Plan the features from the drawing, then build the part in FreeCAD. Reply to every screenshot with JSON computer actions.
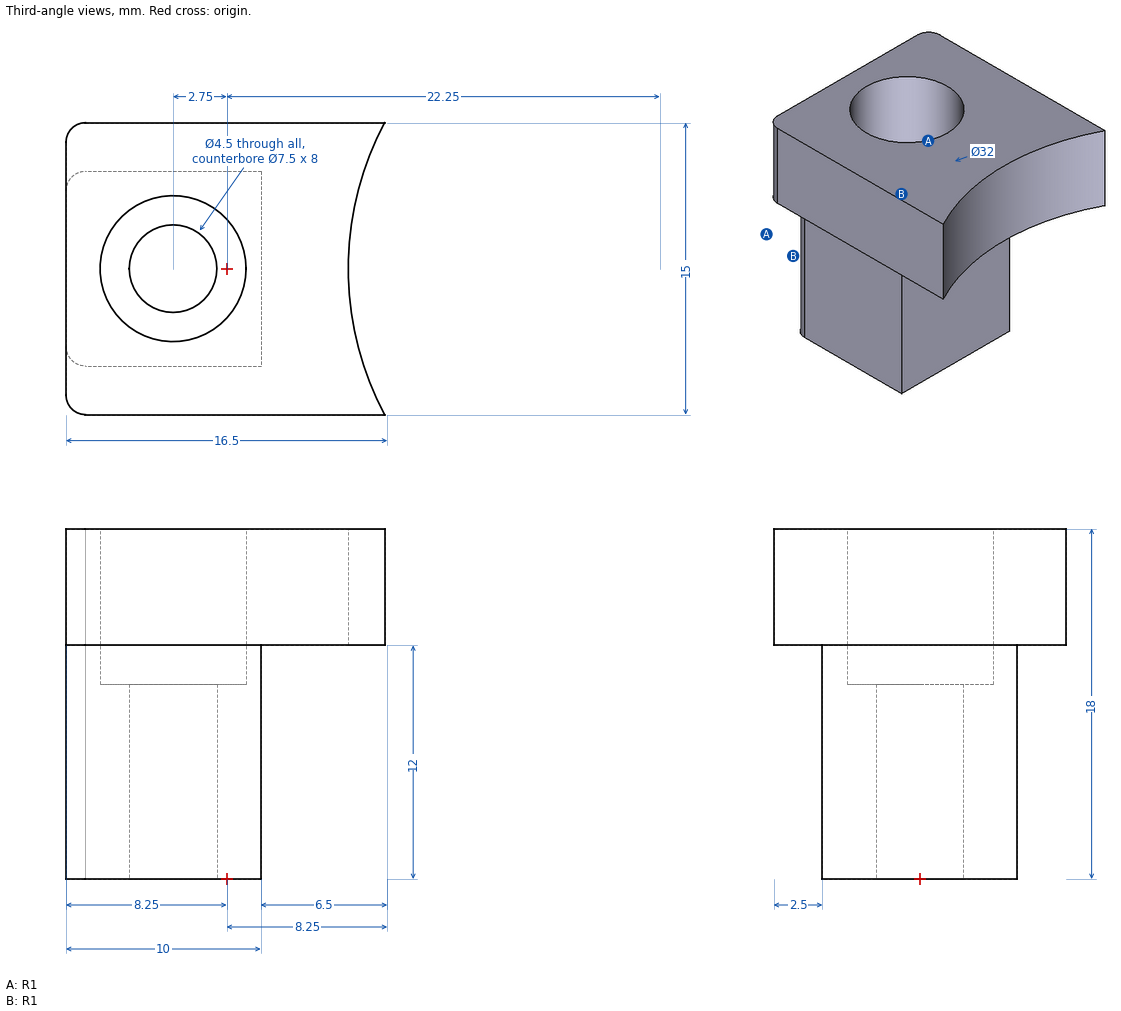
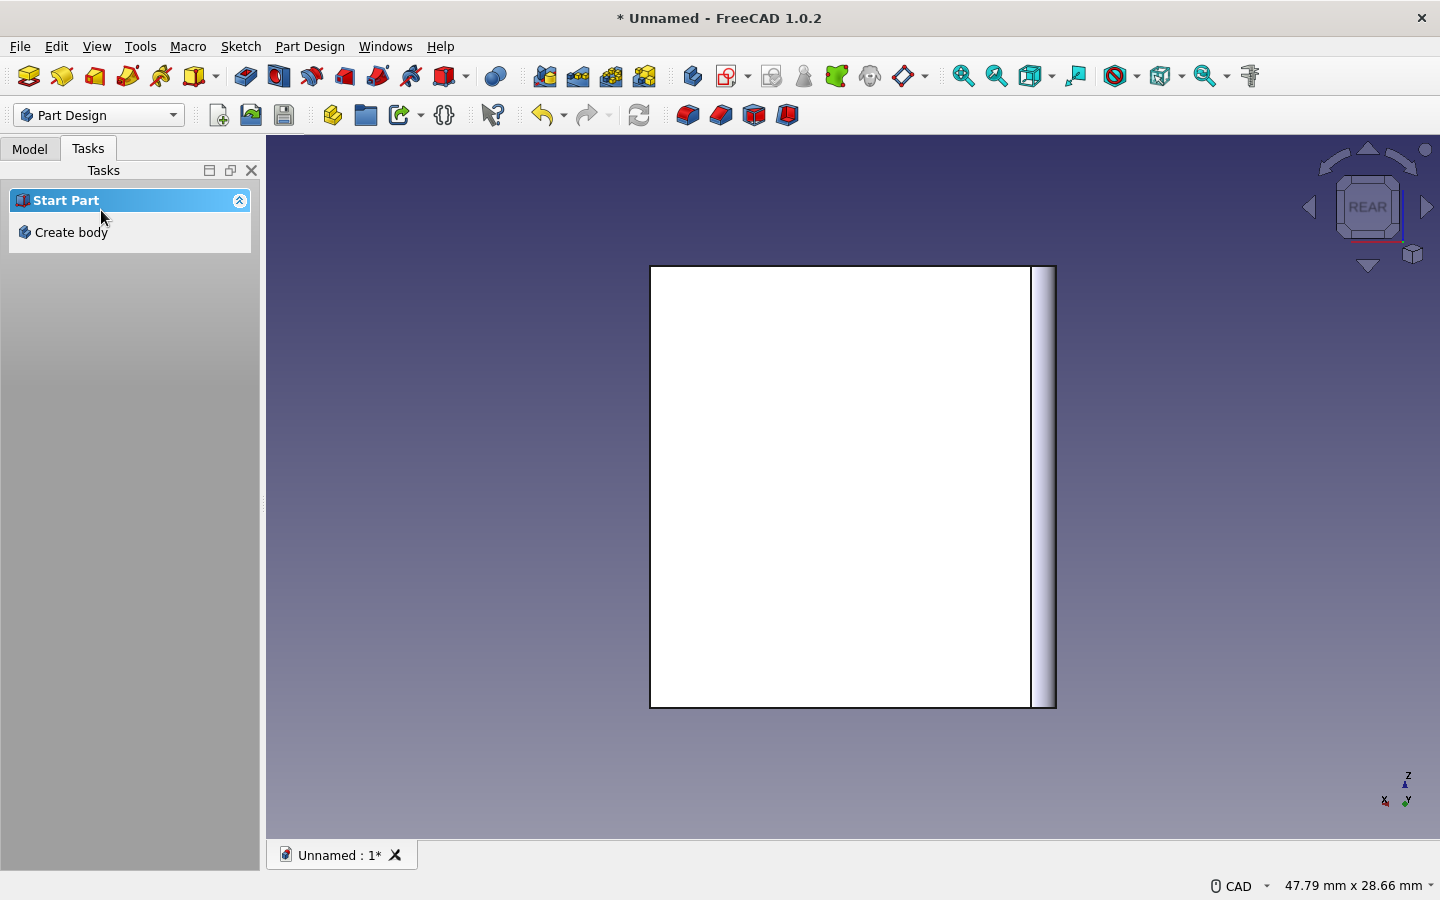
{"action": "key", "text": "0"}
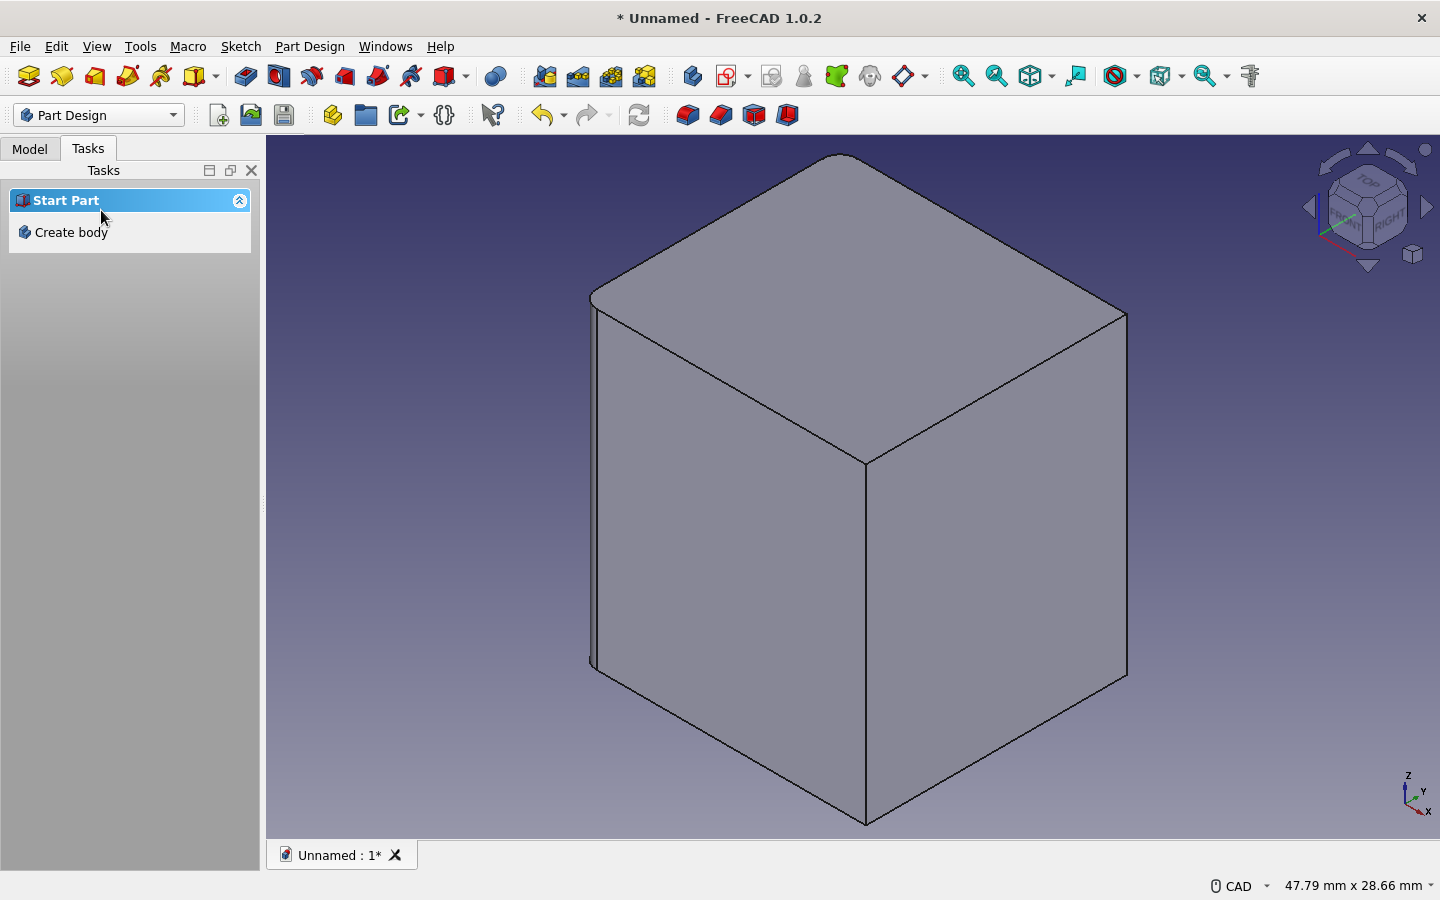
{"action": "left_click", "coordinate": [853, 305]}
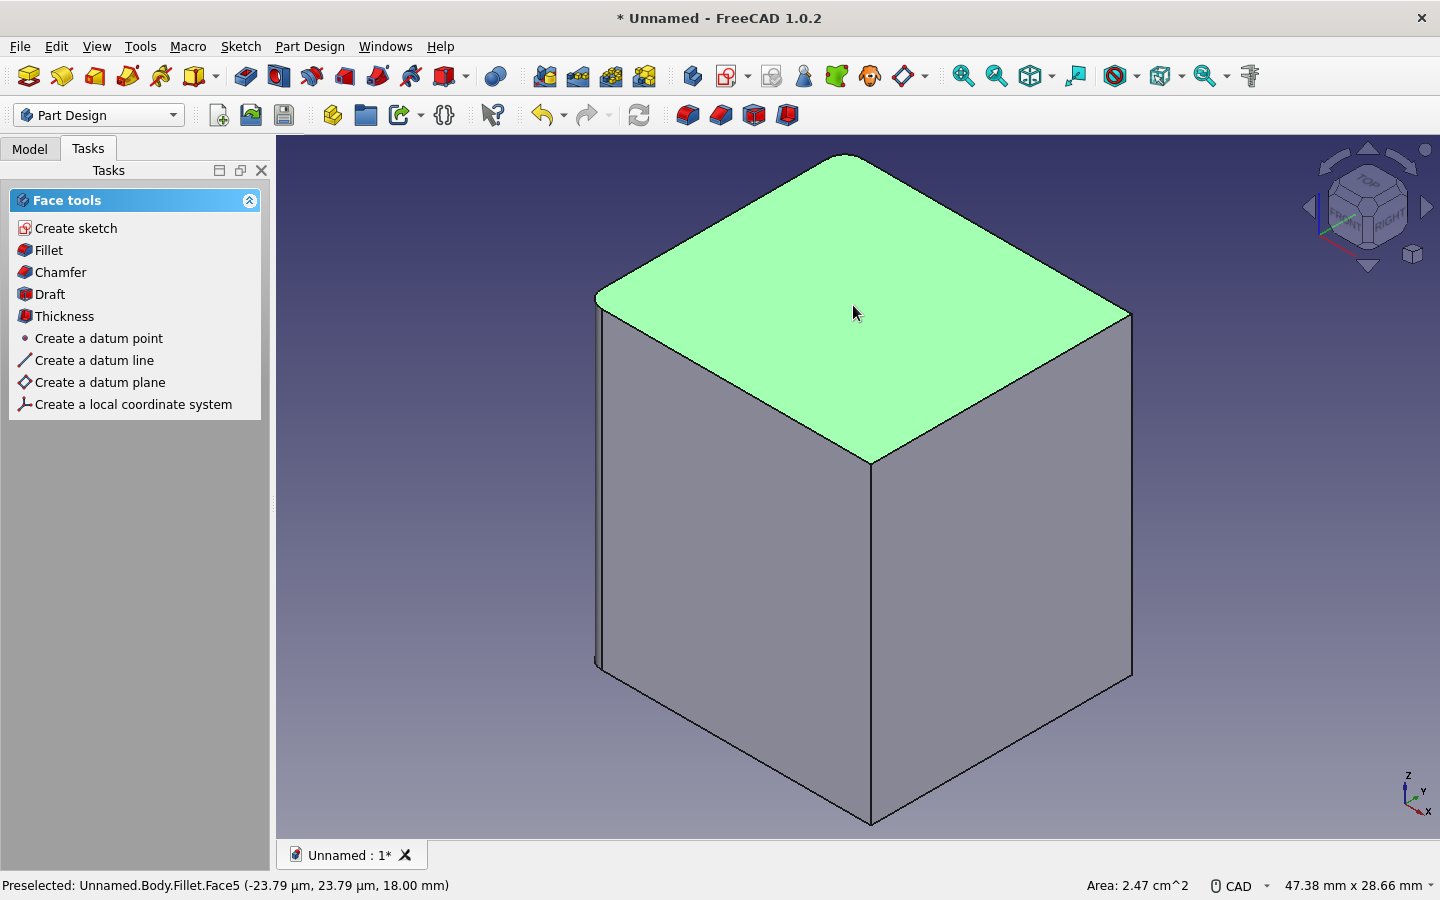
{"action": "left_click", "coordinate": [726, 76]}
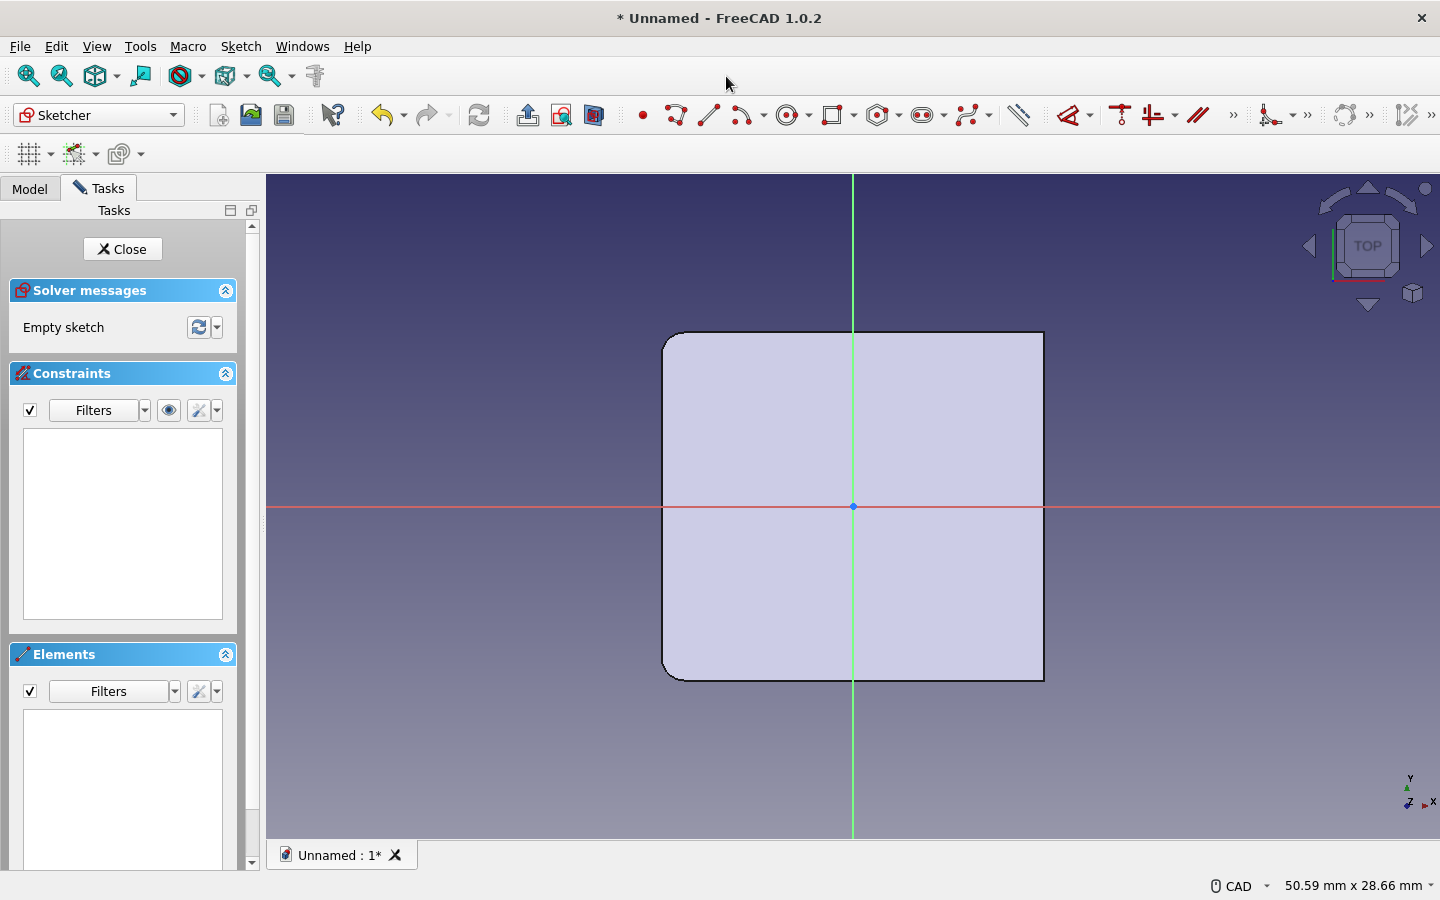
{"action": "scroll", "coordinate": [798, 507], "scroll_direction": "up", "scroll_amount": 7}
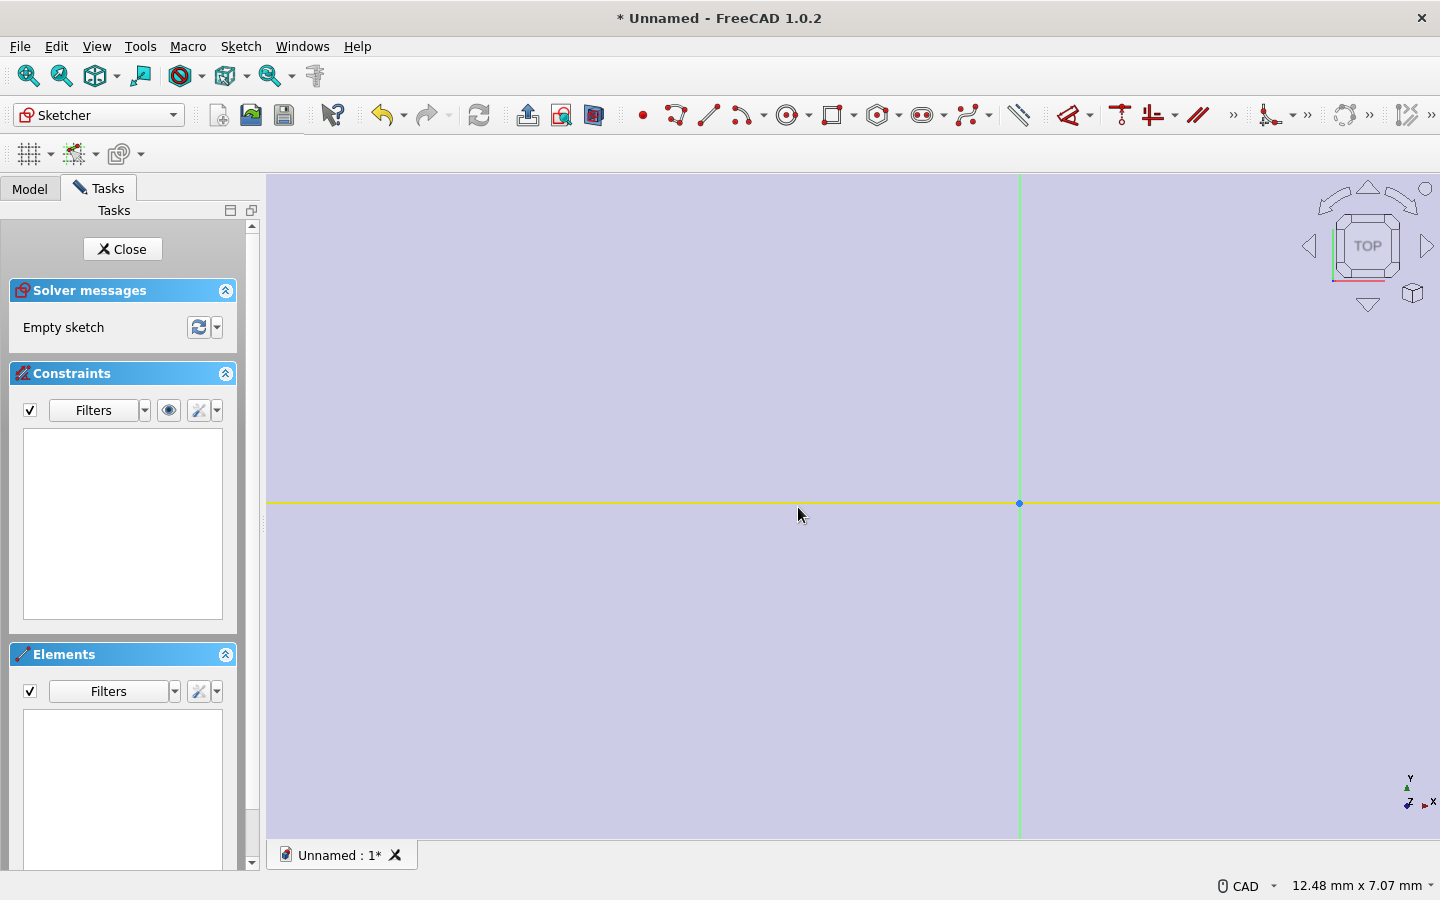
{"action": "key", "text": "g c"}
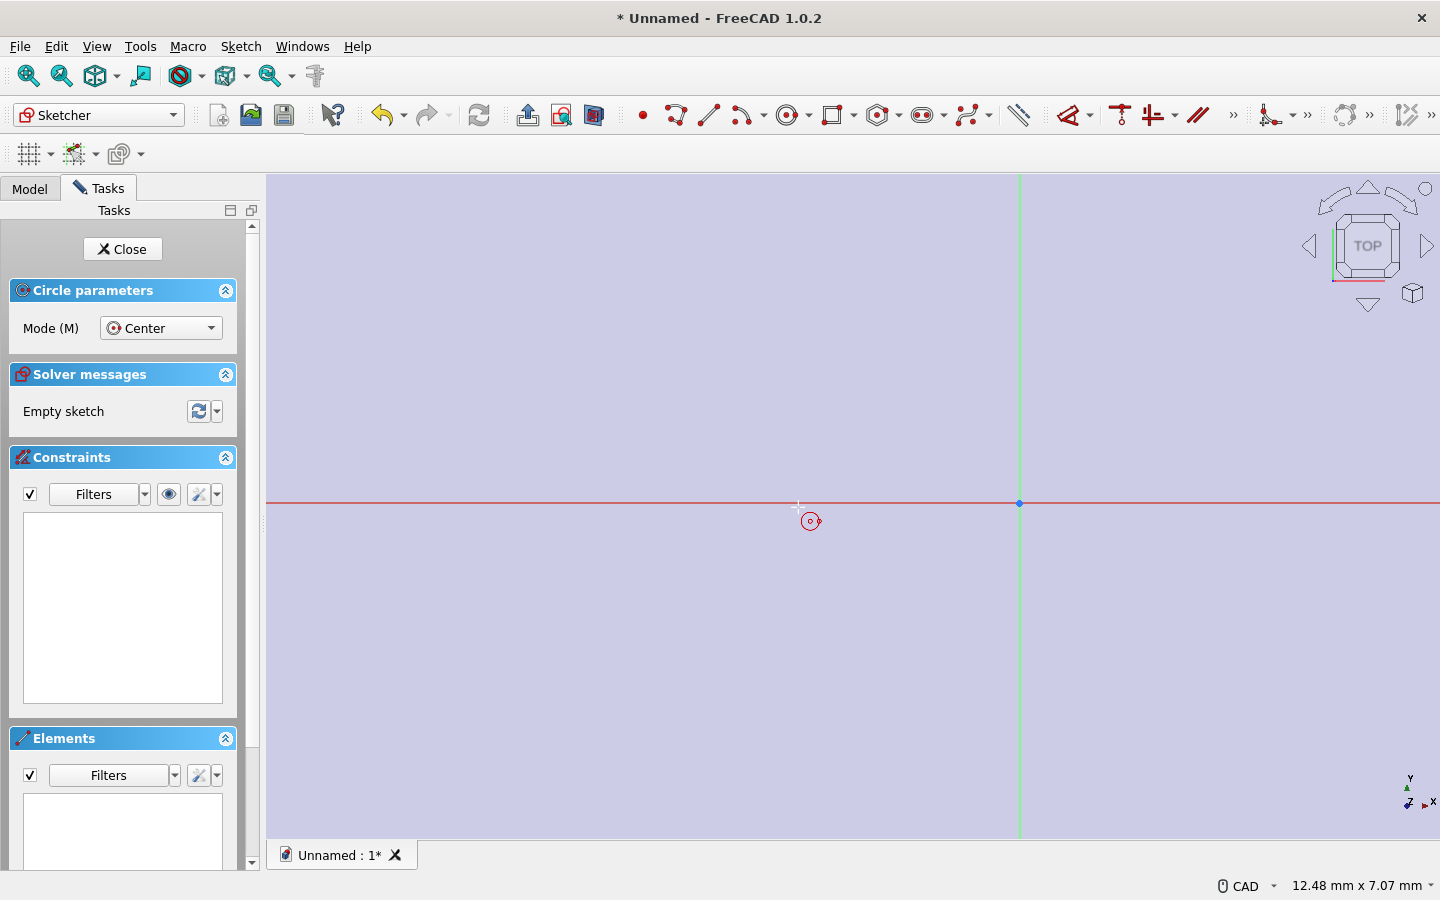
{"action": "left_click", "coordinate": [761, 503]}
{"action": "left_click", "coordinate": [911, 354]}
{"action": "key", "text": "Escape"}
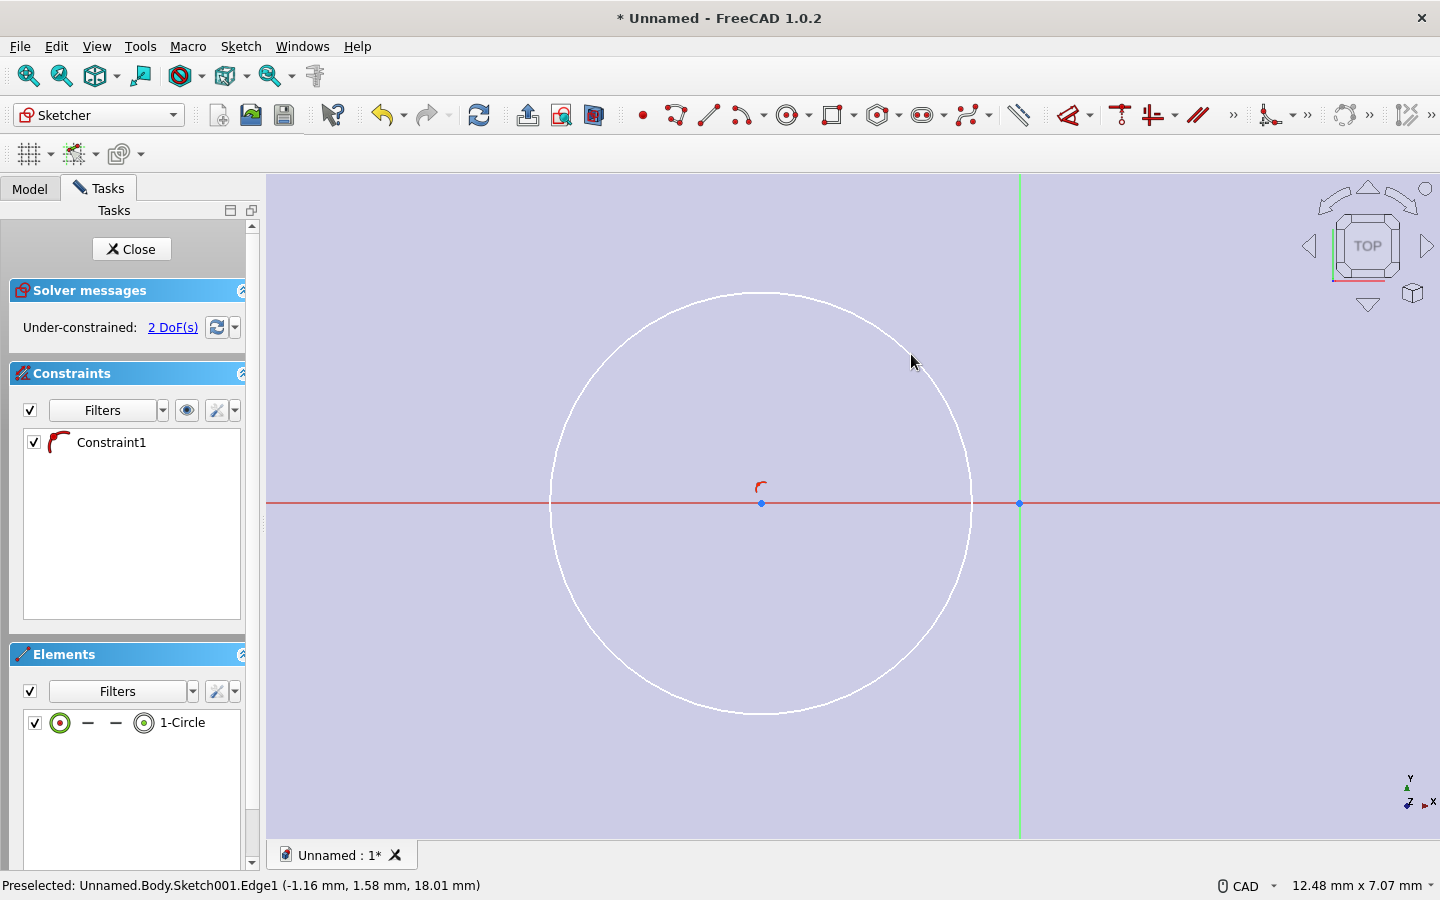
{"action": "left_click", "coordinate": [1068, 116]}